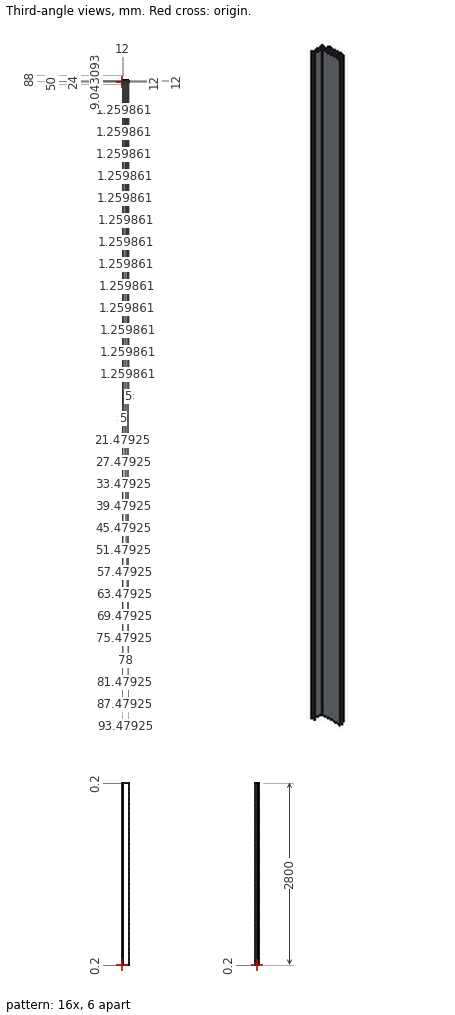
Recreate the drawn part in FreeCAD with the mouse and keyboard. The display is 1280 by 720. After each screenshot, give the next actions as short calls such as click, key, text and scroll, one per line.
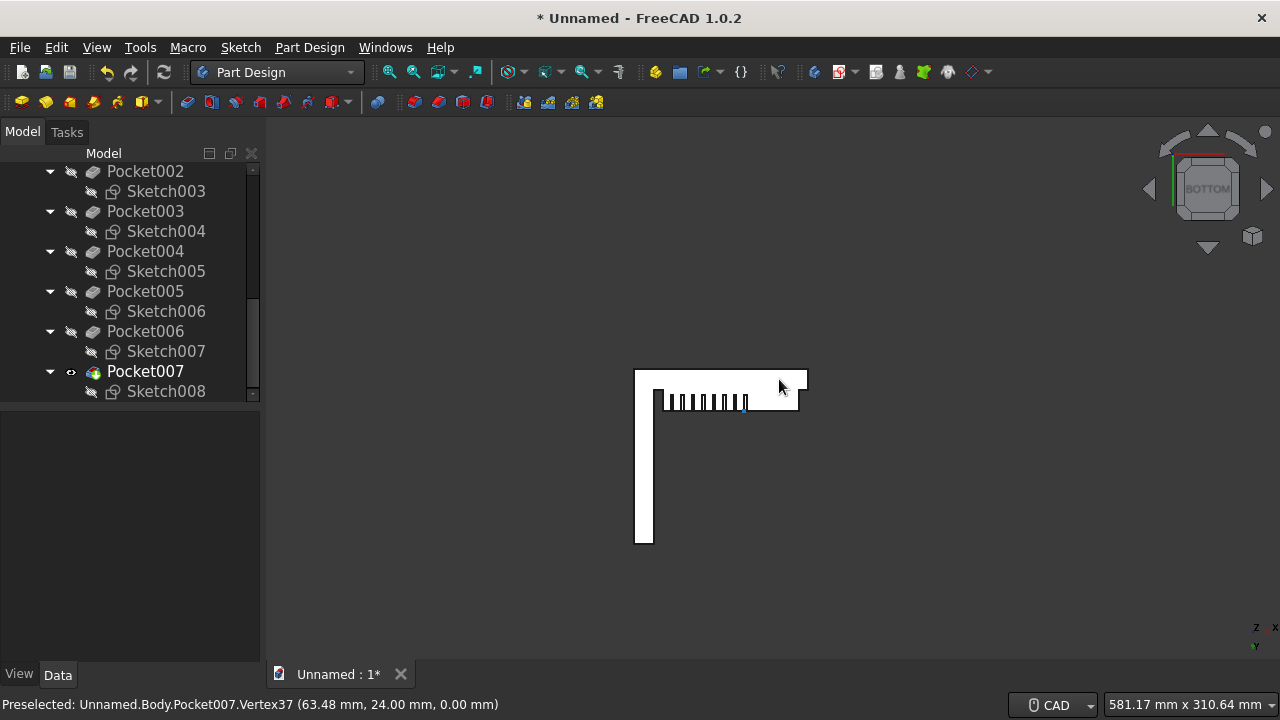
click(771, 381)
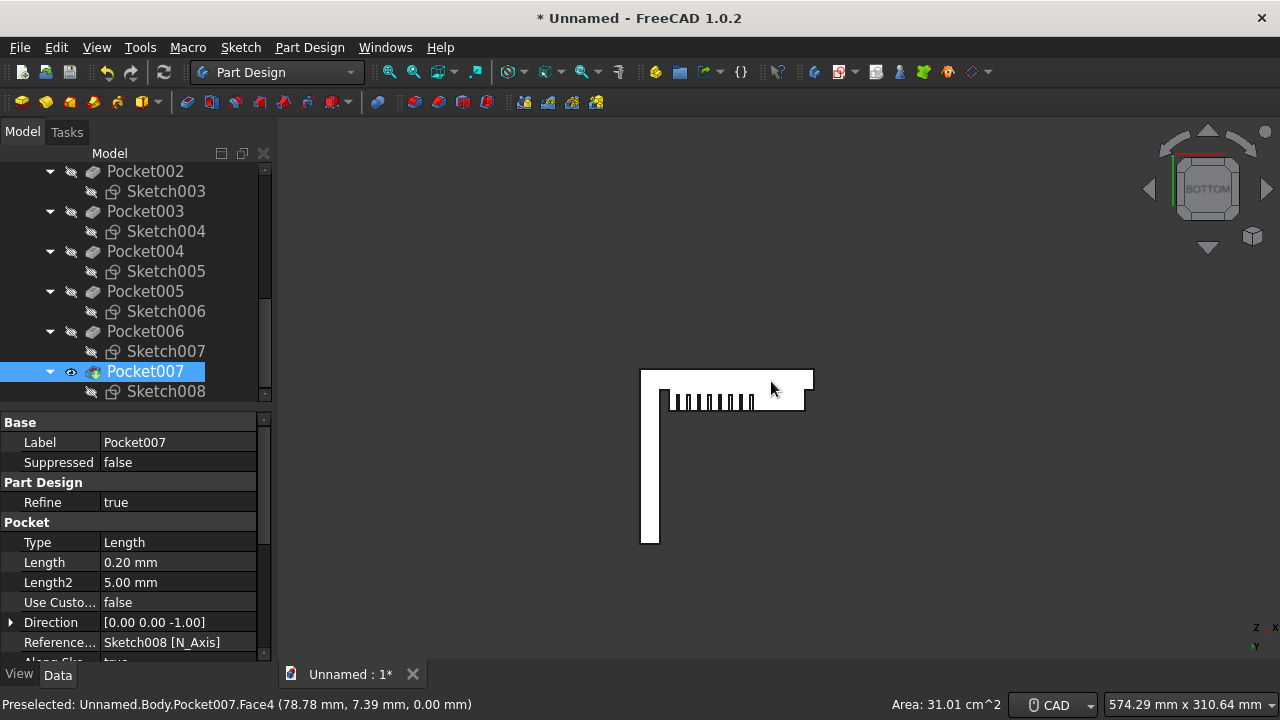
click(840, 72)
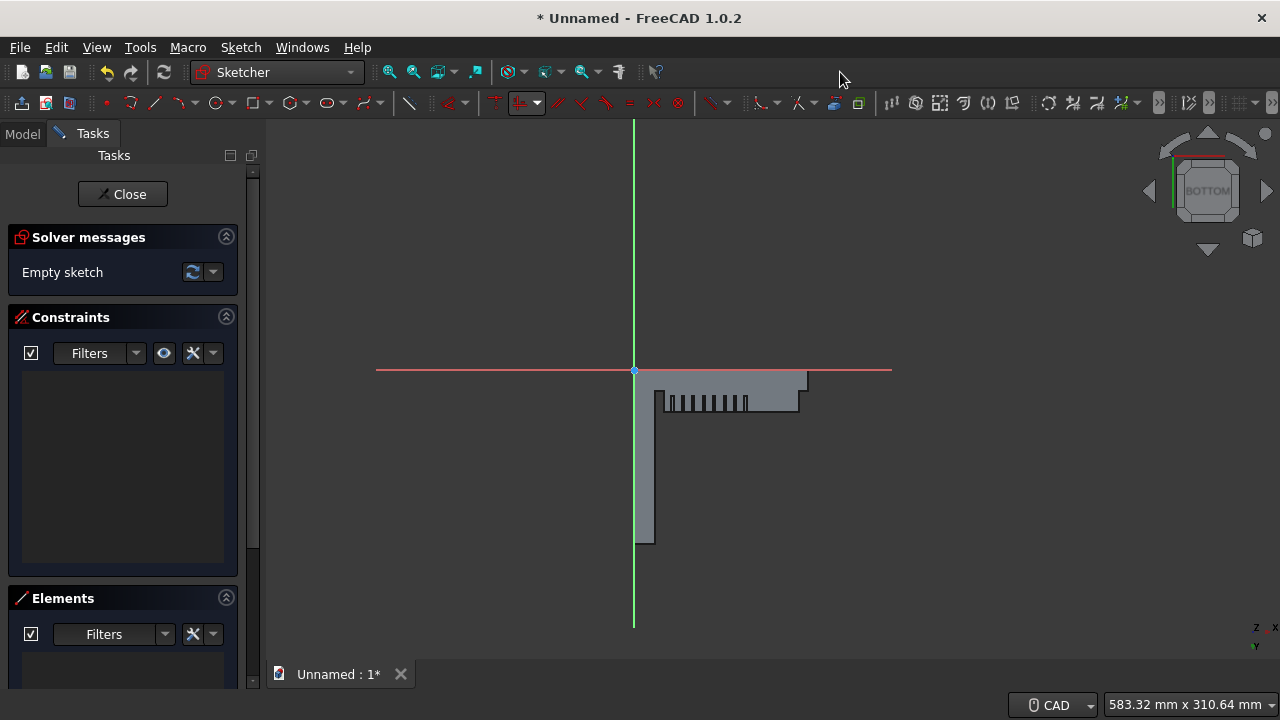
scroll(759, 405, up, 15)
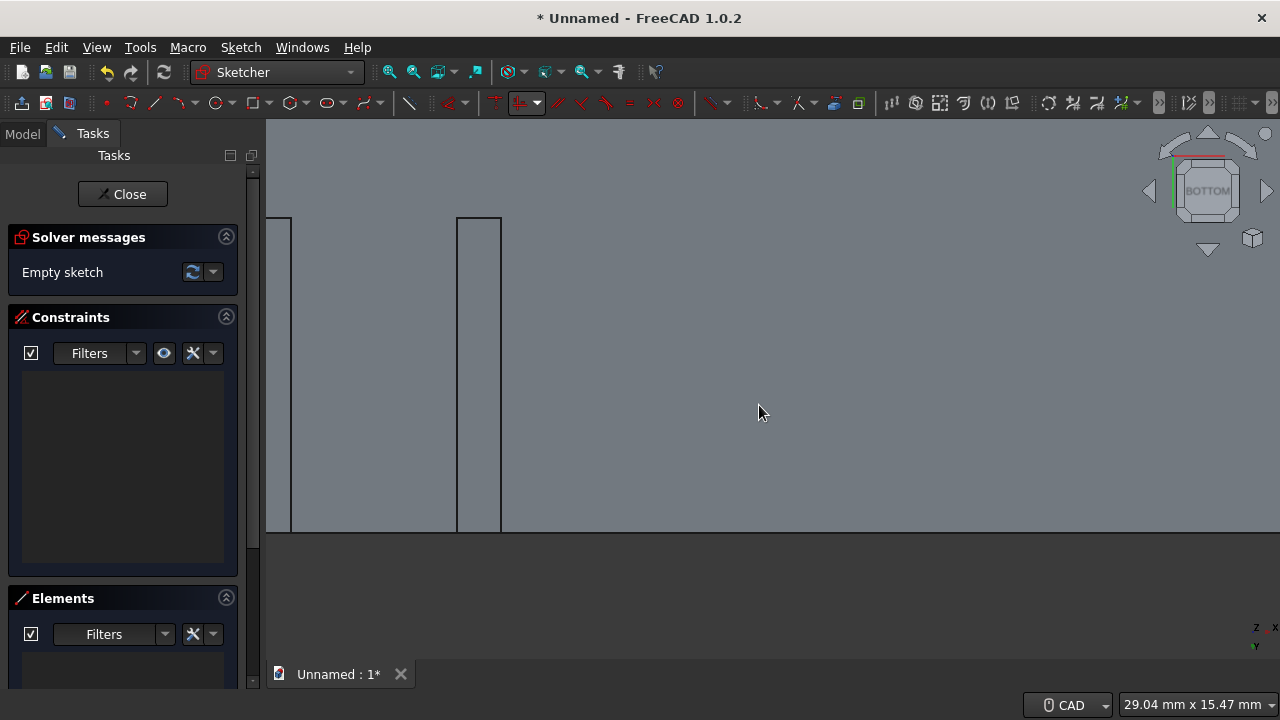
click(254, 104)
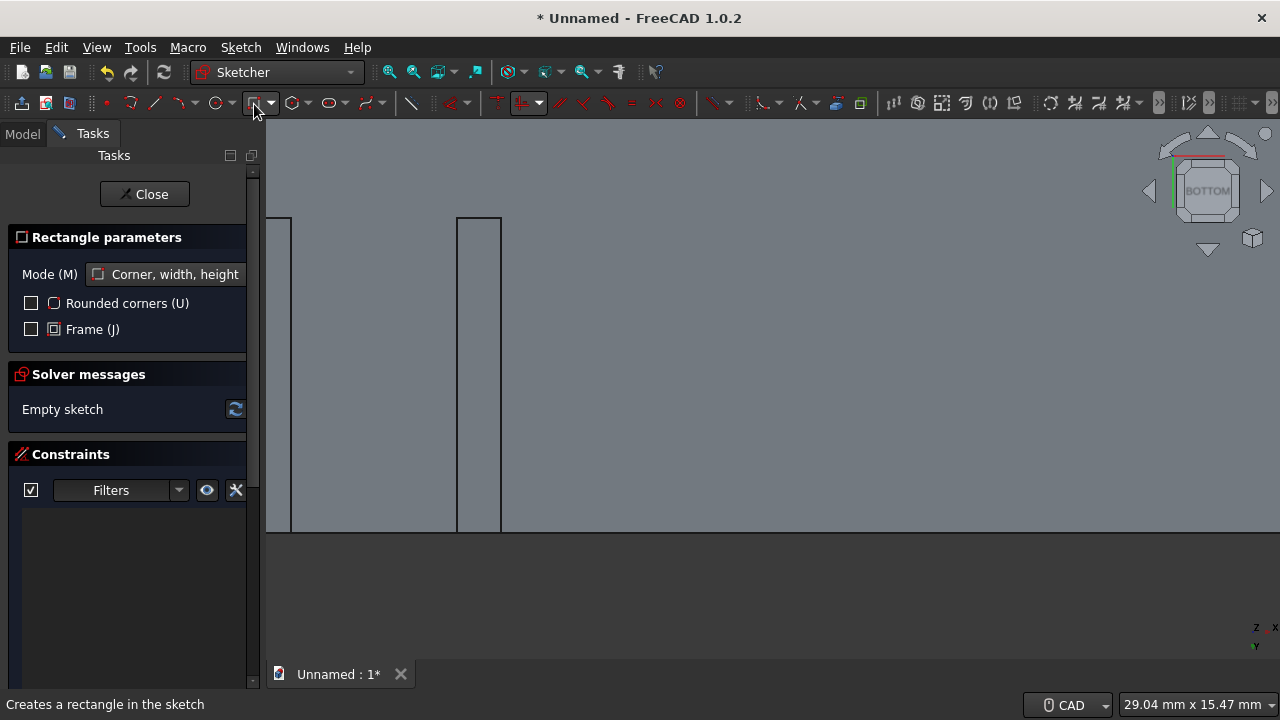
click(666, 218)
move(710, 533)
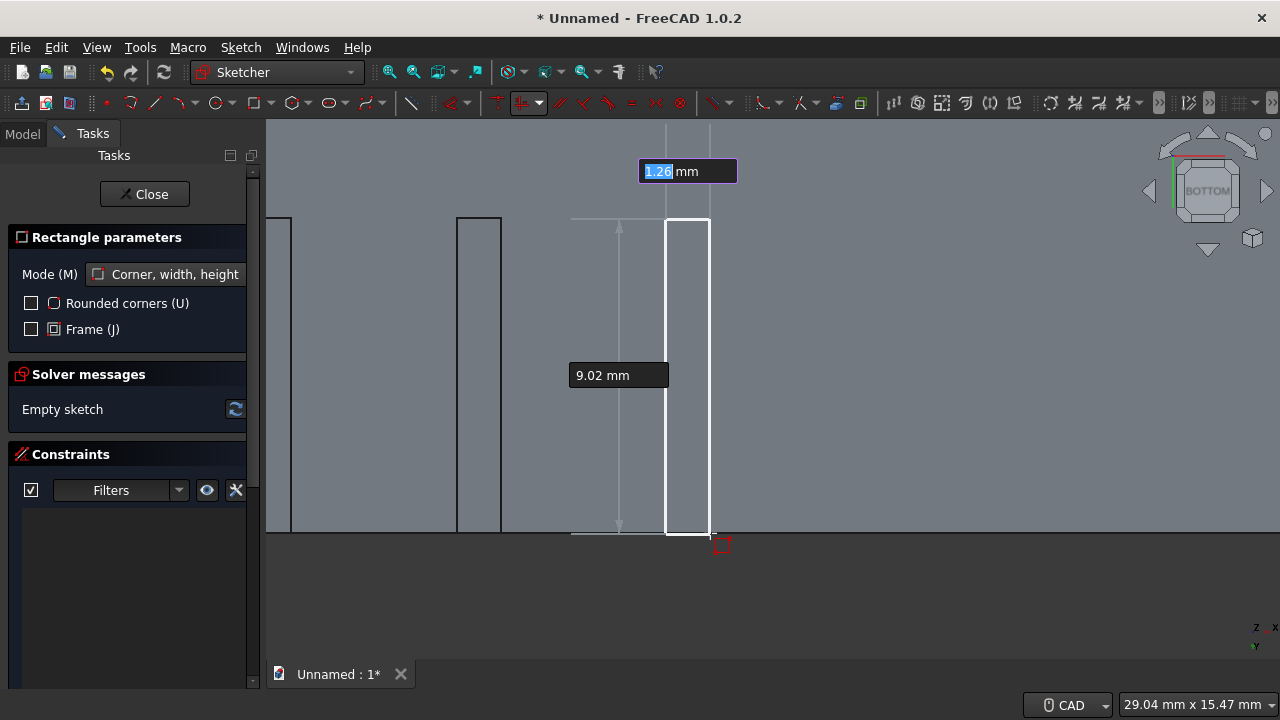
text(1.259861)
key(Tab)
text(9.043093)
key(Return)
key(Escape)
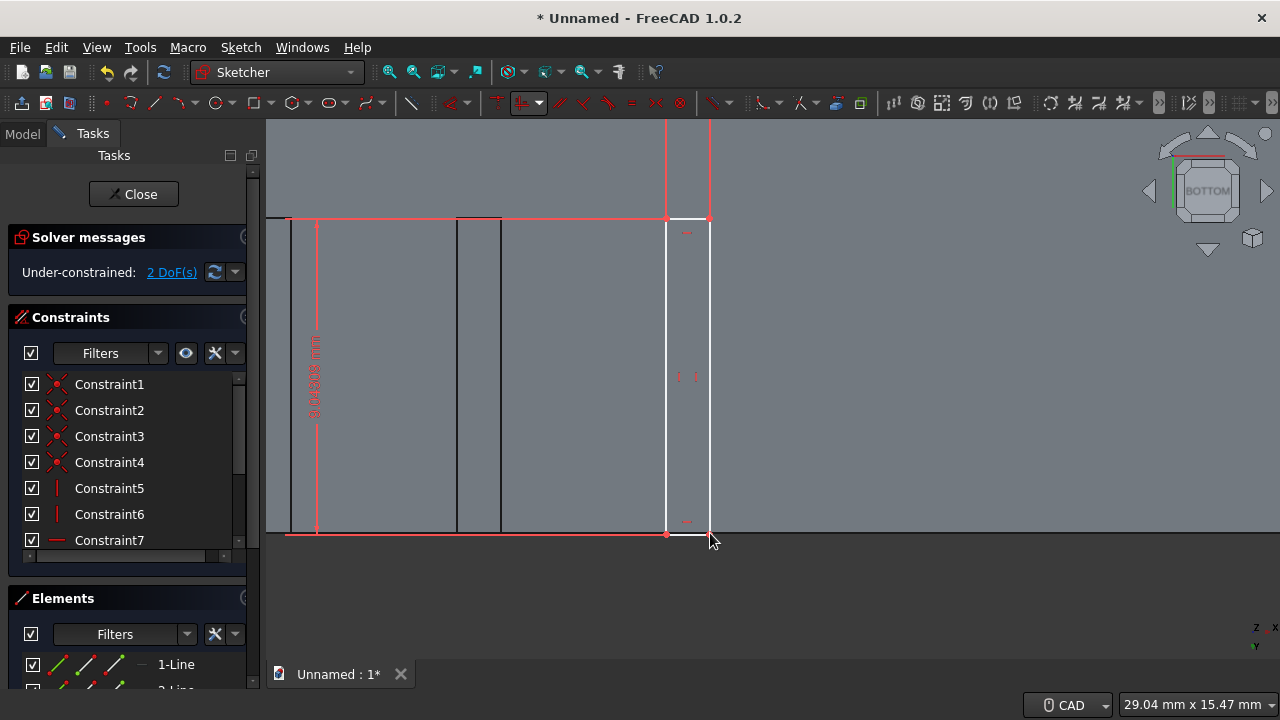
click(450, 104)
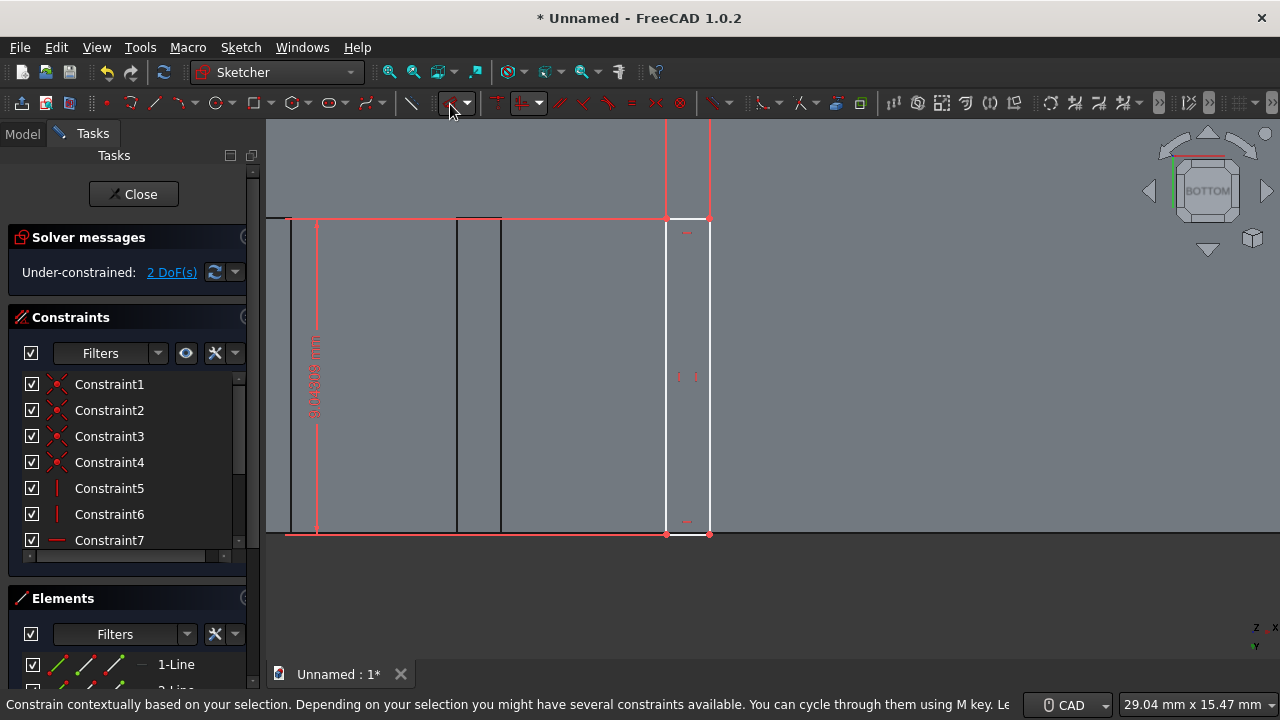
click(666, 535)
click(700, 205)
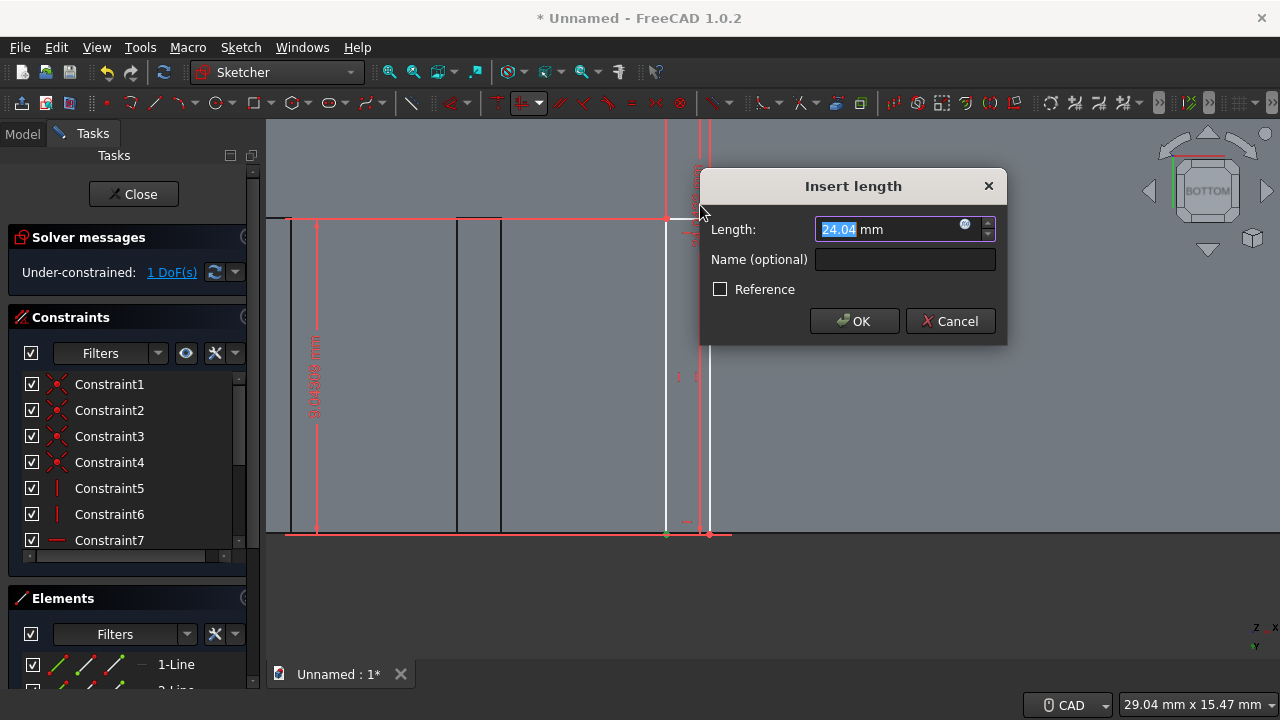
text(24)
key(Return)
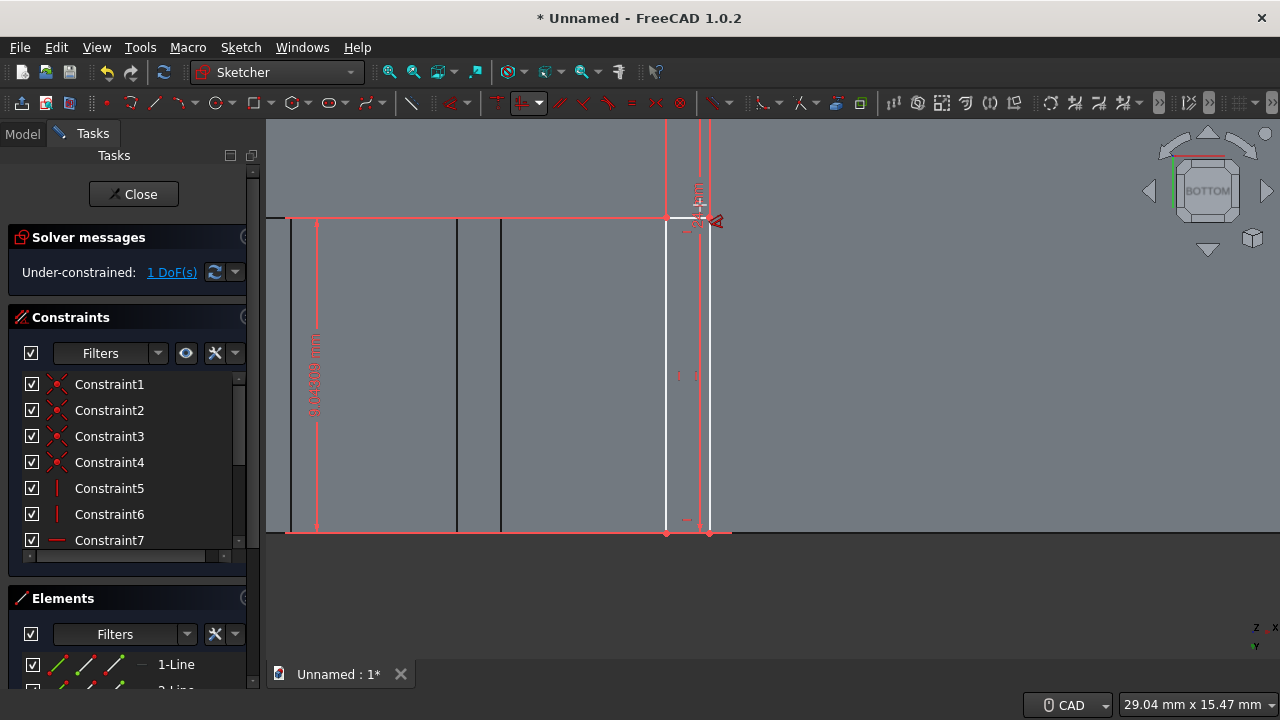
click(666, 218)
click(480, 252)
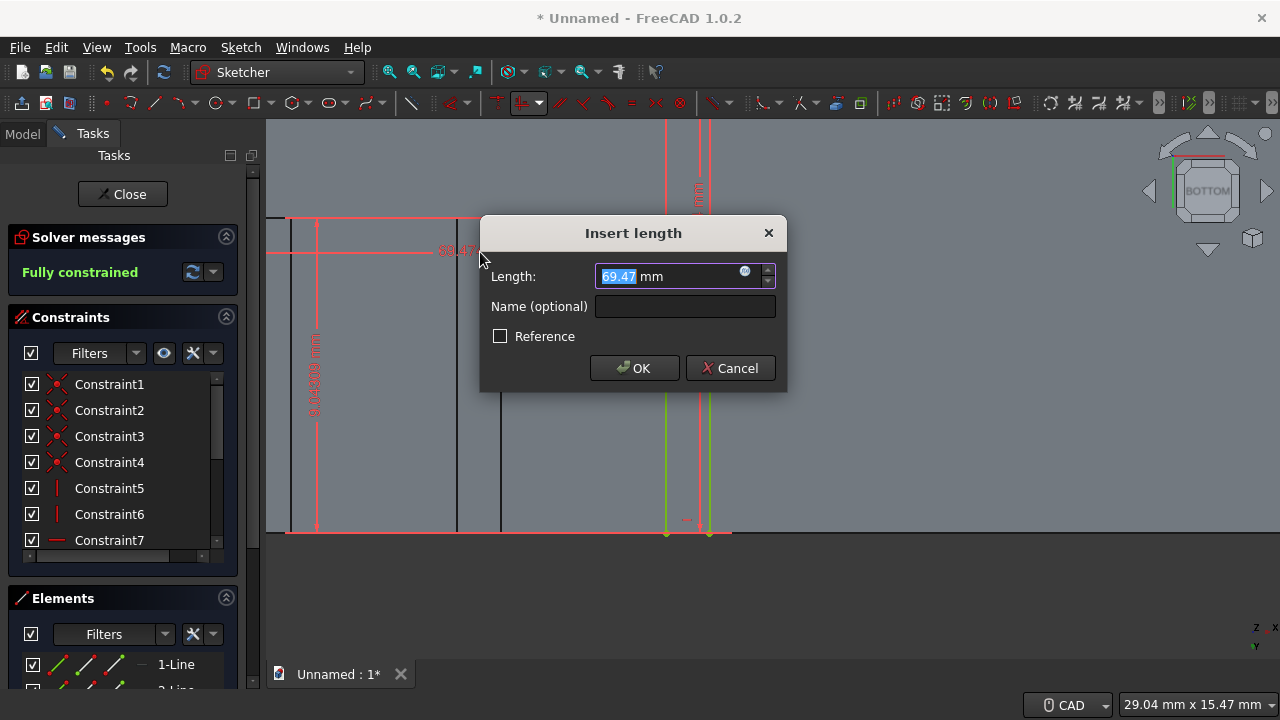
text(69.47925)
key(Return)
key(Escape)